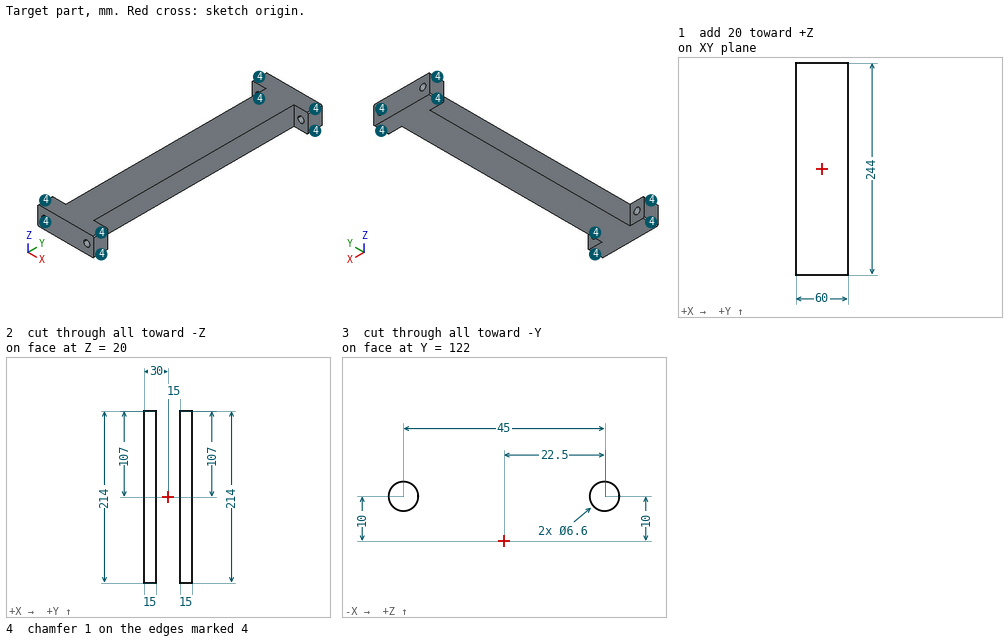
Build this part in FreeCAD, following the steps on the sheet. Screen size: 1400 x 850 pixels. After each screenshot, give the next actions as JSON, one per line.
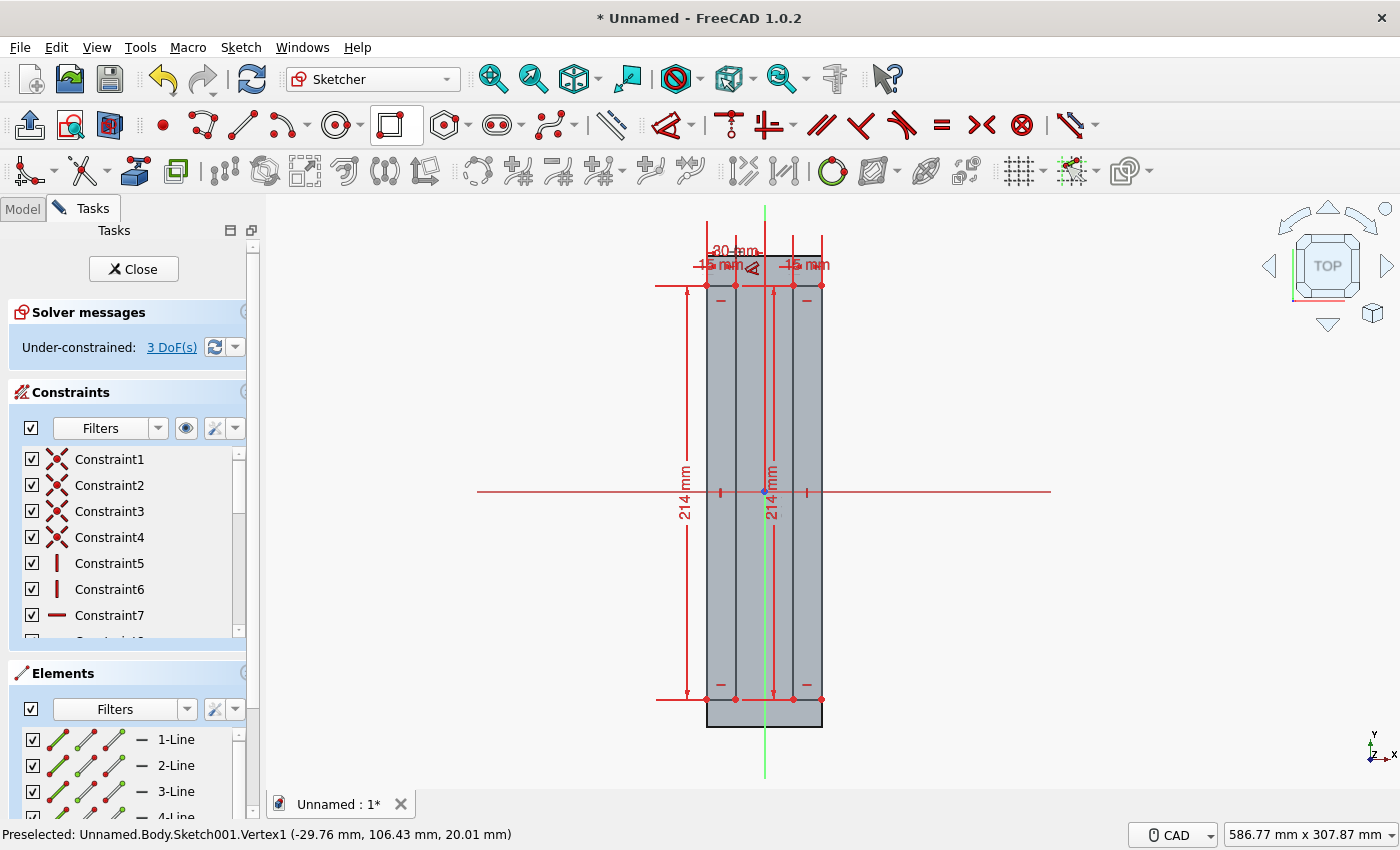
{"action": "scroll", "coordinate": [793, 286], "scroll_direction": "up", "scroll_amount": 2}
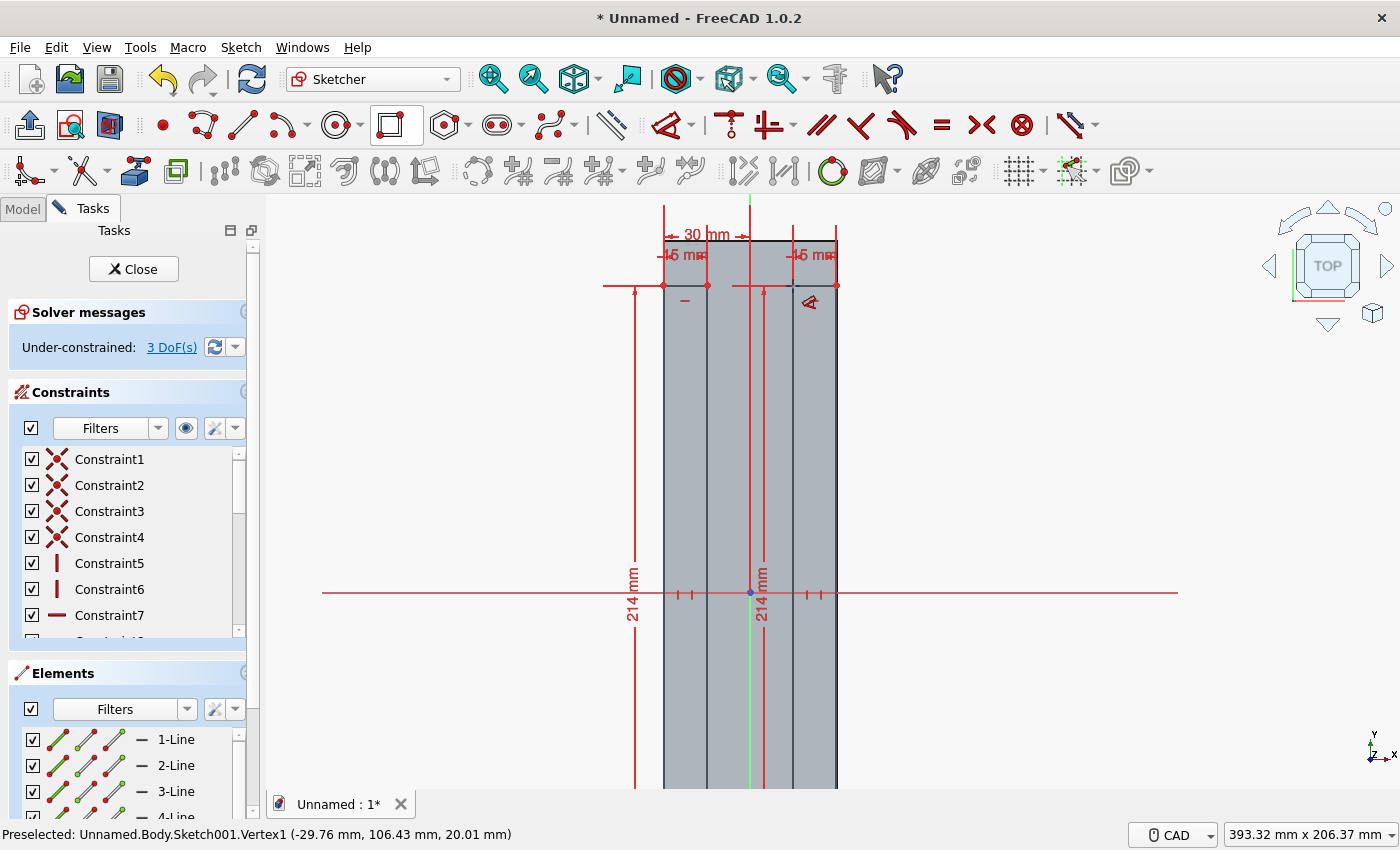
{"action": "left_click", "coordinate": [793, 286]}
{"action": "left_click", "coordinate": [781, 252]}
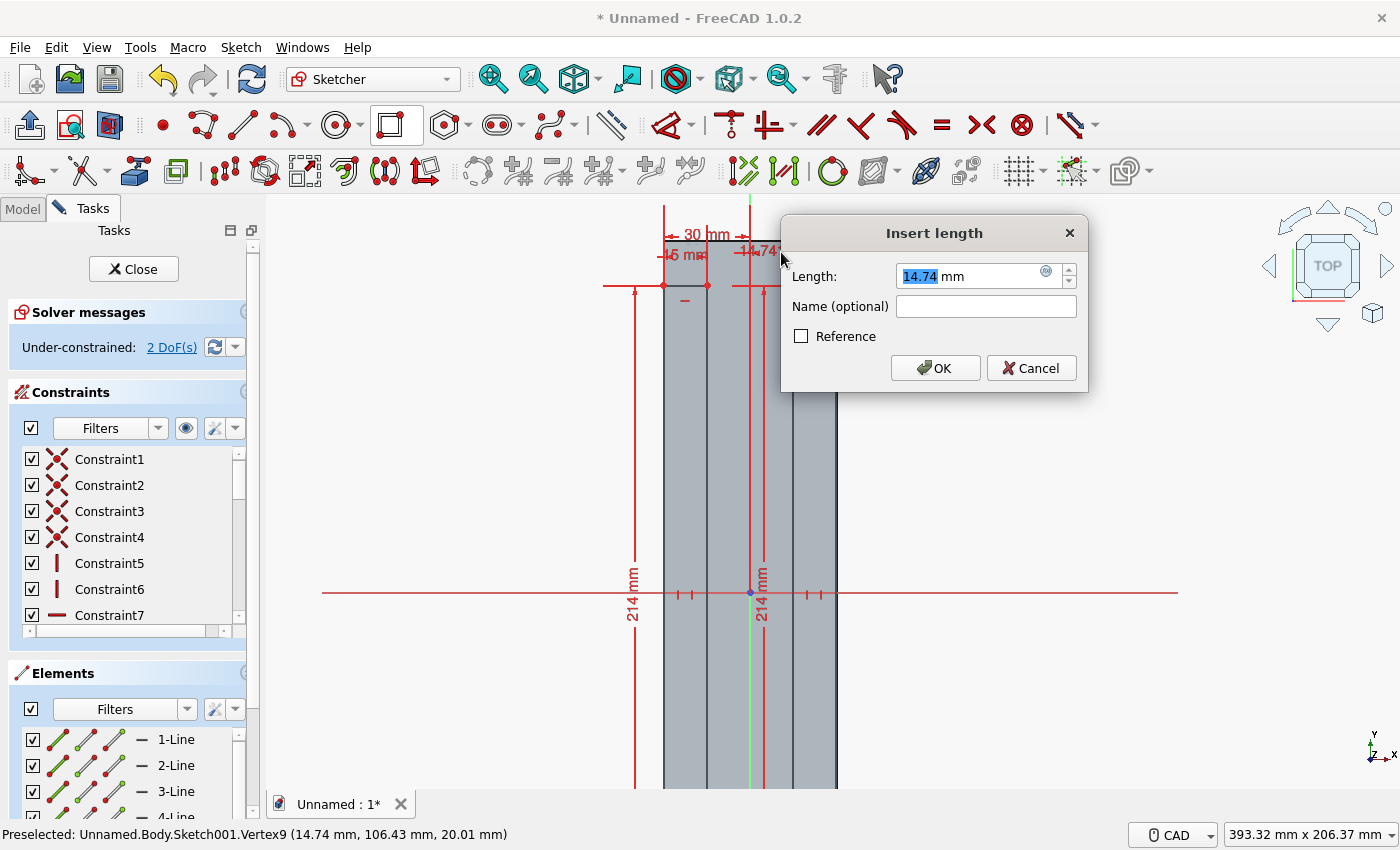
{"action": "type", "text": "15"}
{"action": "key", "text": "Return"}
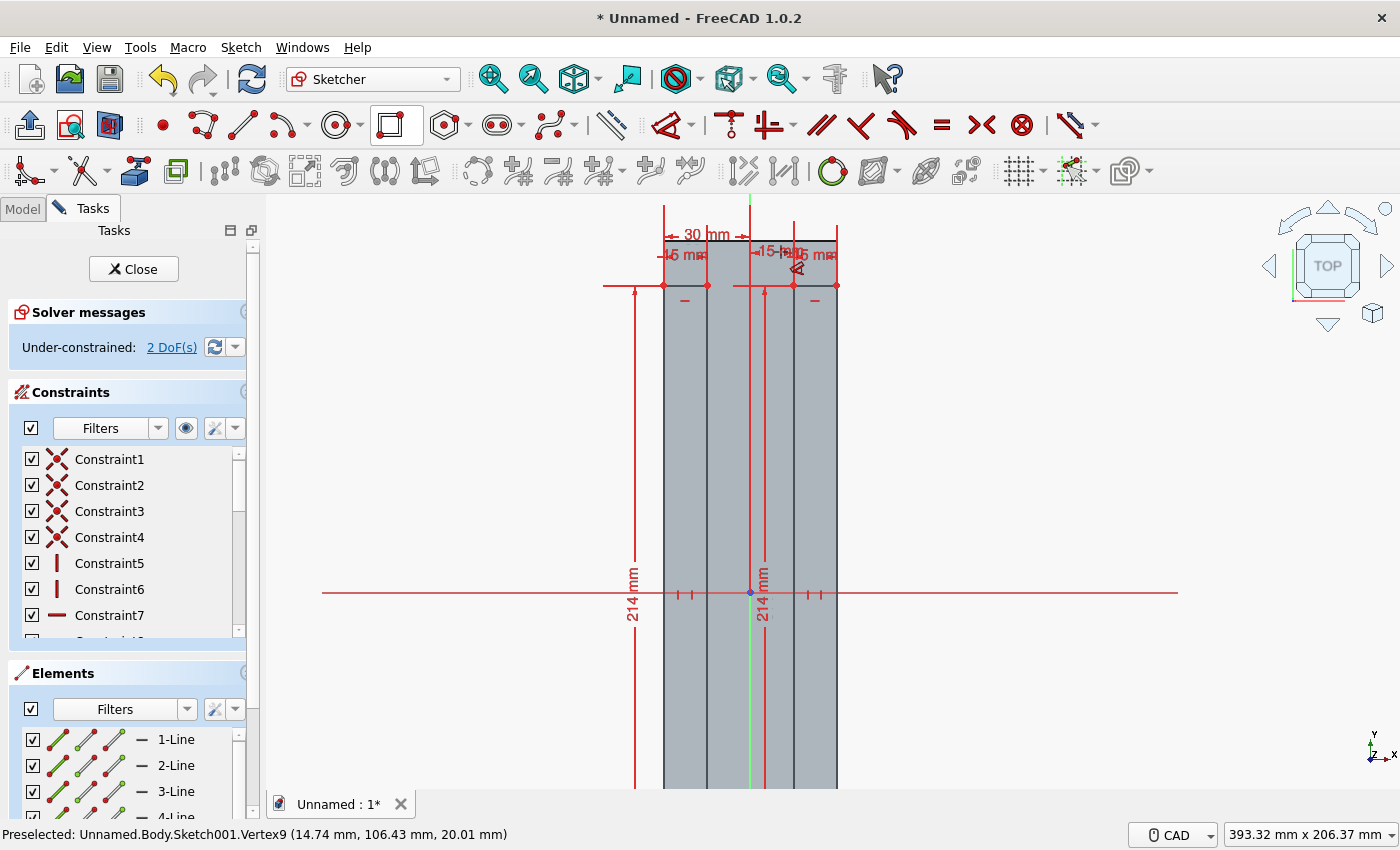
{"action": "left_click", "coordinate": [664, 286]}
{"action": "left_click", "coordinate": [630, 439]}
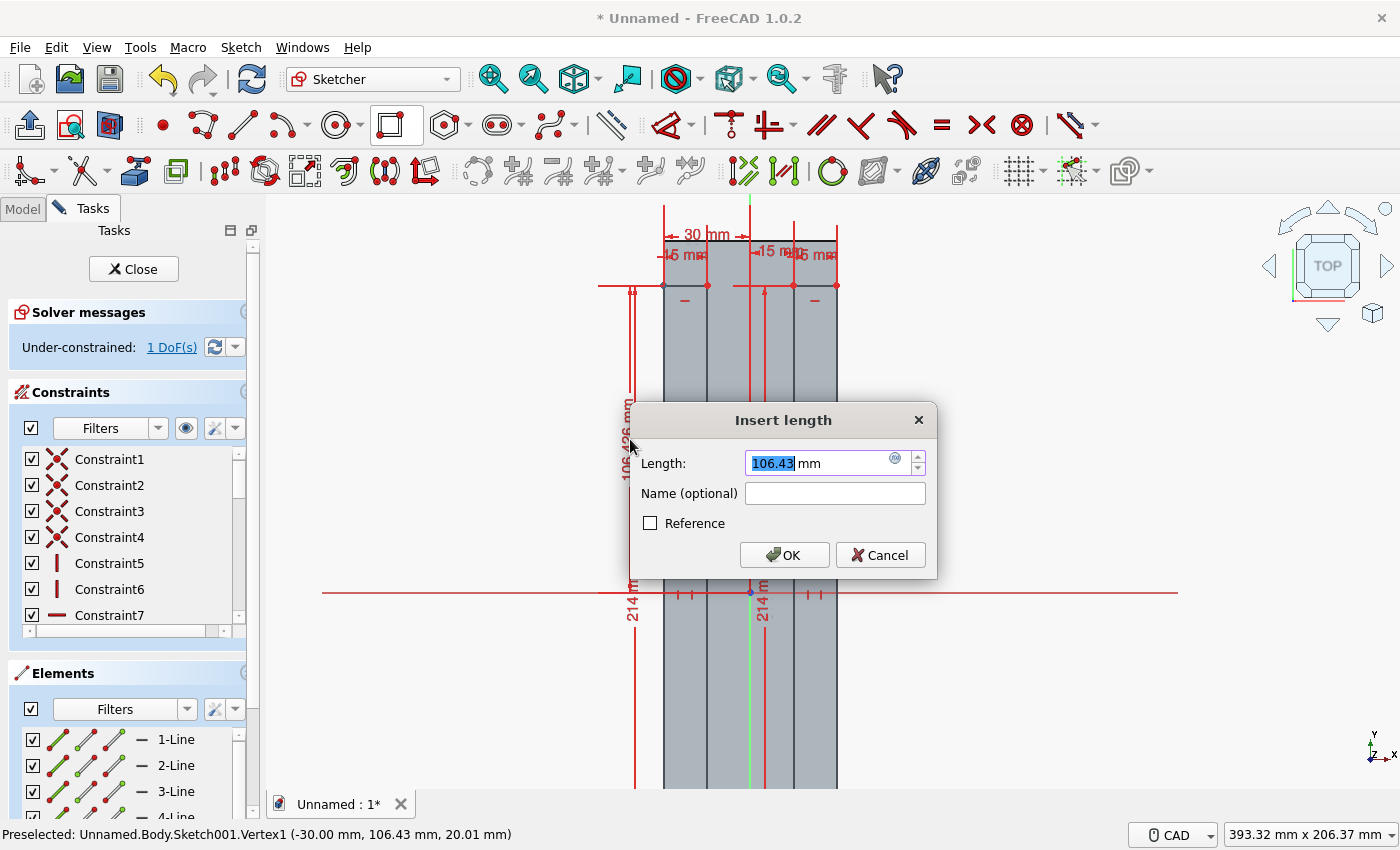
{"action": "type", "text": "107"}
{"action": "key", "text": "Return"}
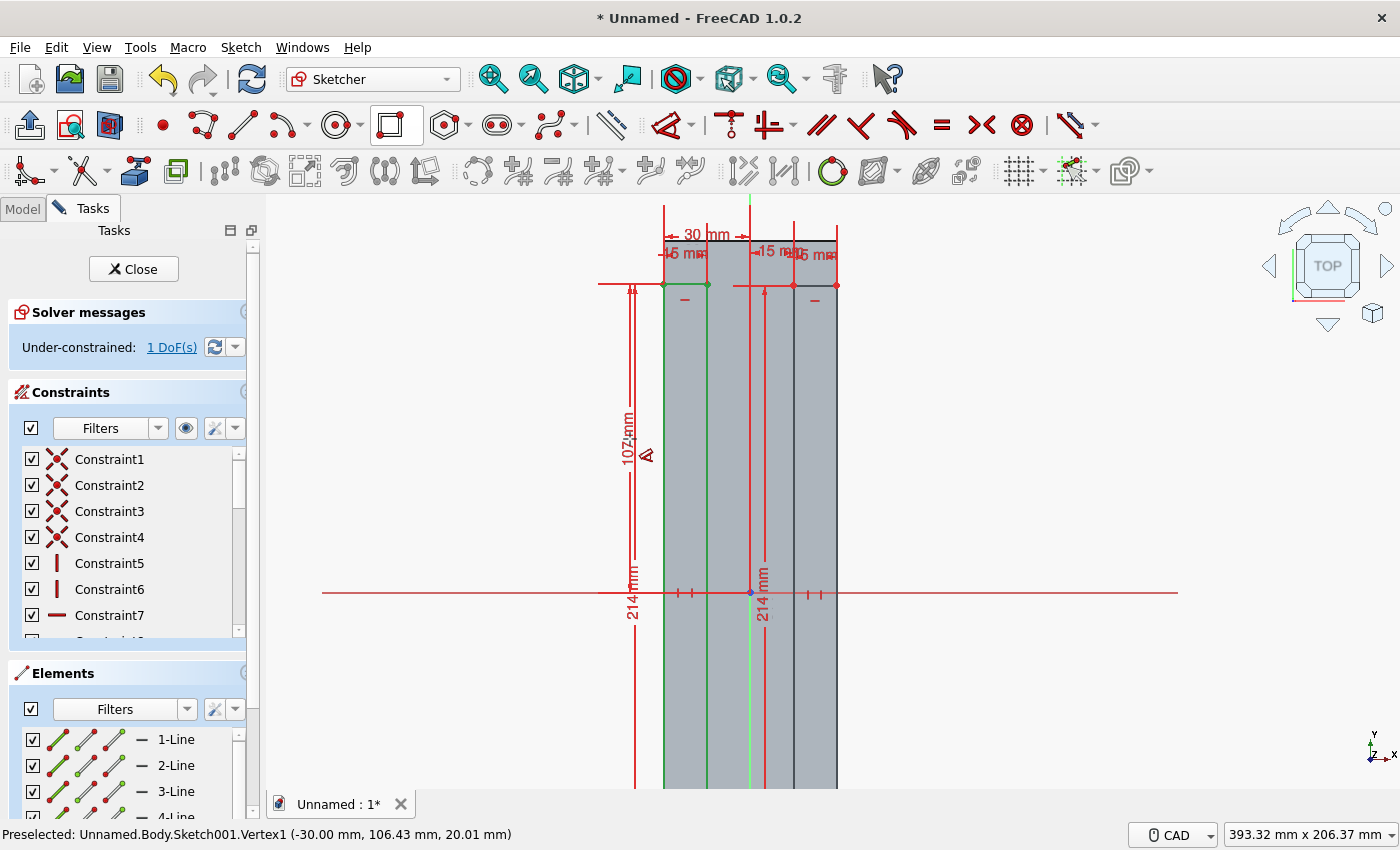
{"action": "left_click", "coordinate": [794, 286]}
{"action": "left_click", "coordinate": [852, 439]}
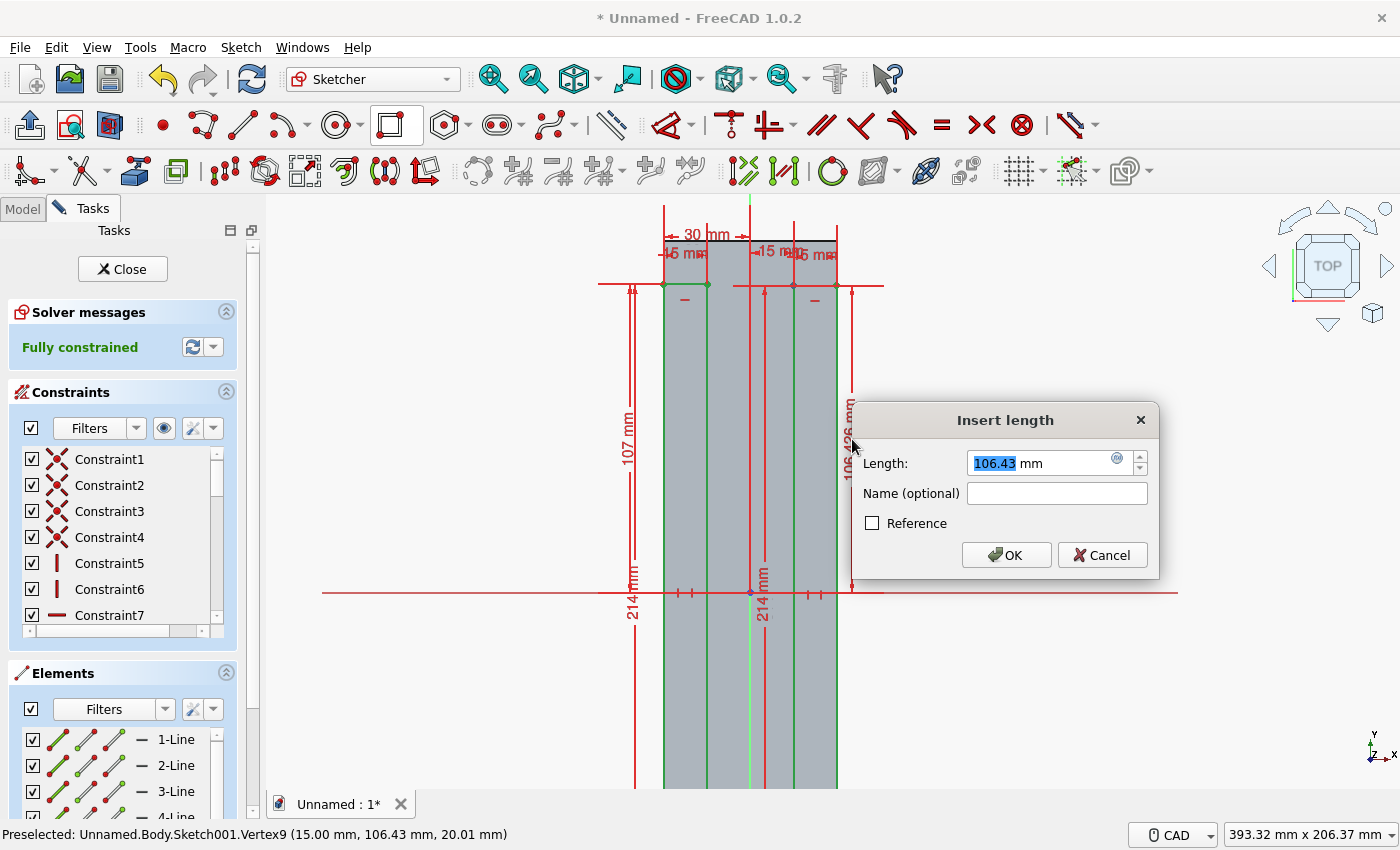
{"action": "type", "text": "107"}
{"action": "key", "text": "Return"}
{"action": "key", "text": "Escape"}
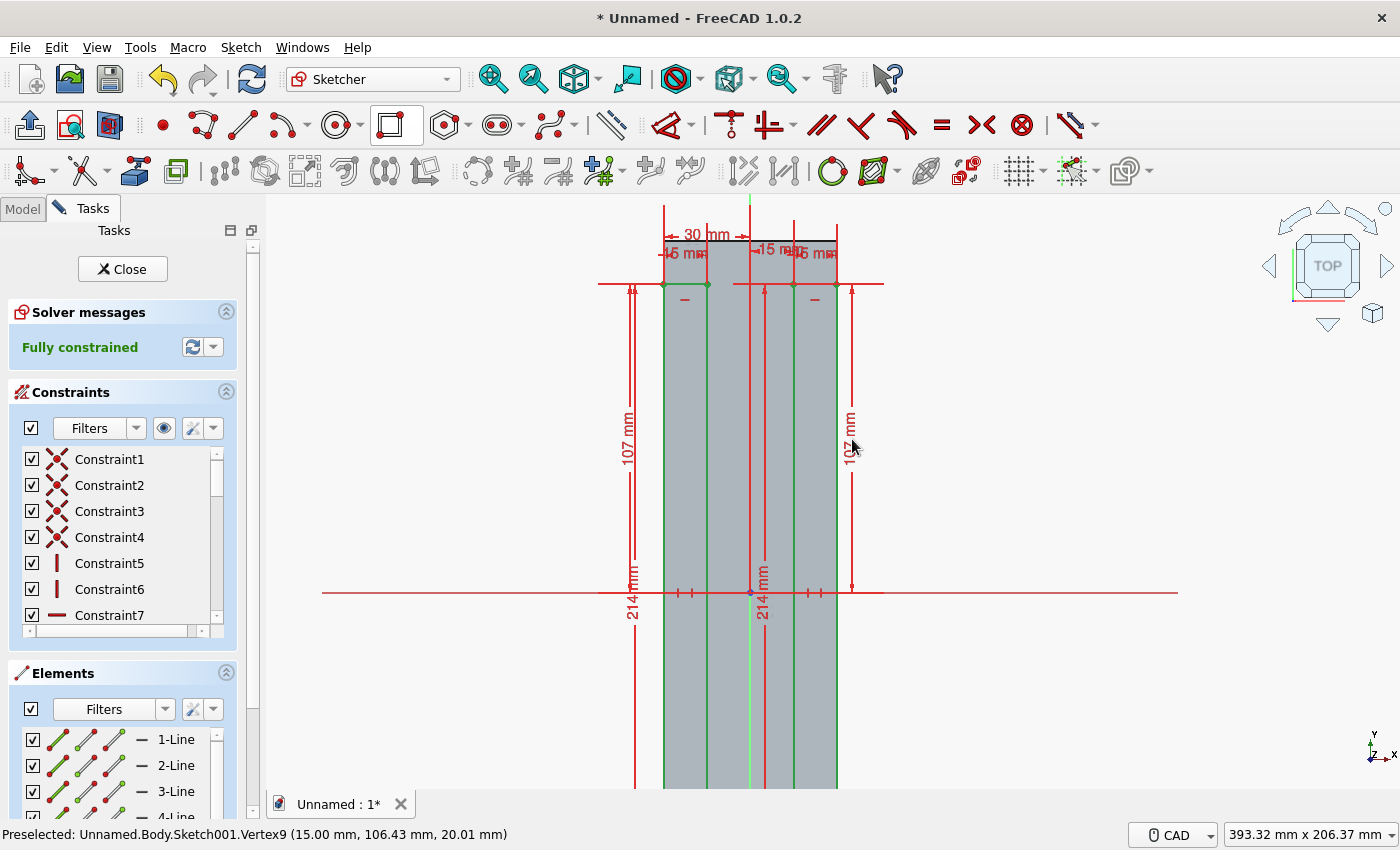
{"action": "left_click", "coordinate": [123, 269]}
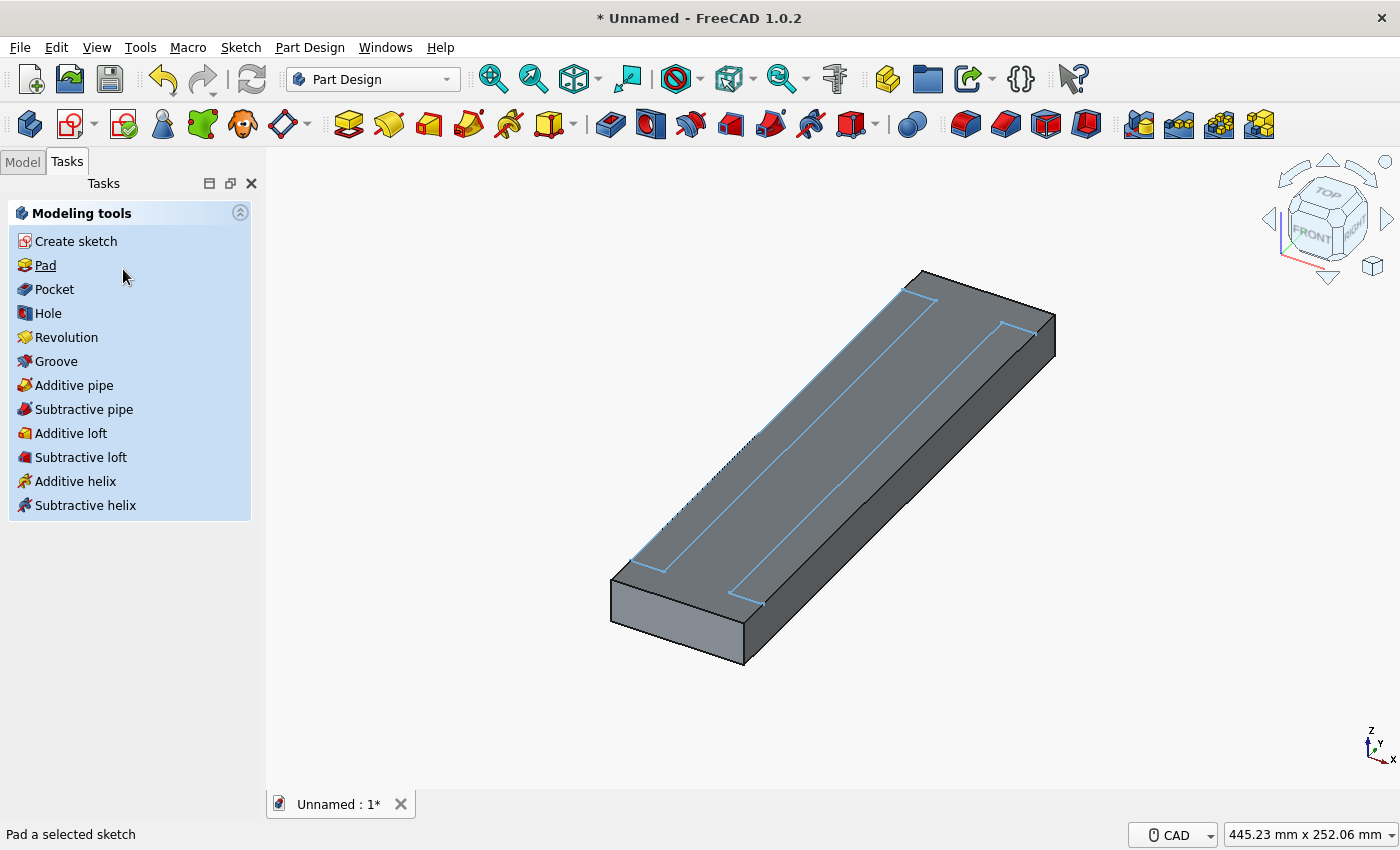
{"action": "left_click", "coordinate": [612, 124]}